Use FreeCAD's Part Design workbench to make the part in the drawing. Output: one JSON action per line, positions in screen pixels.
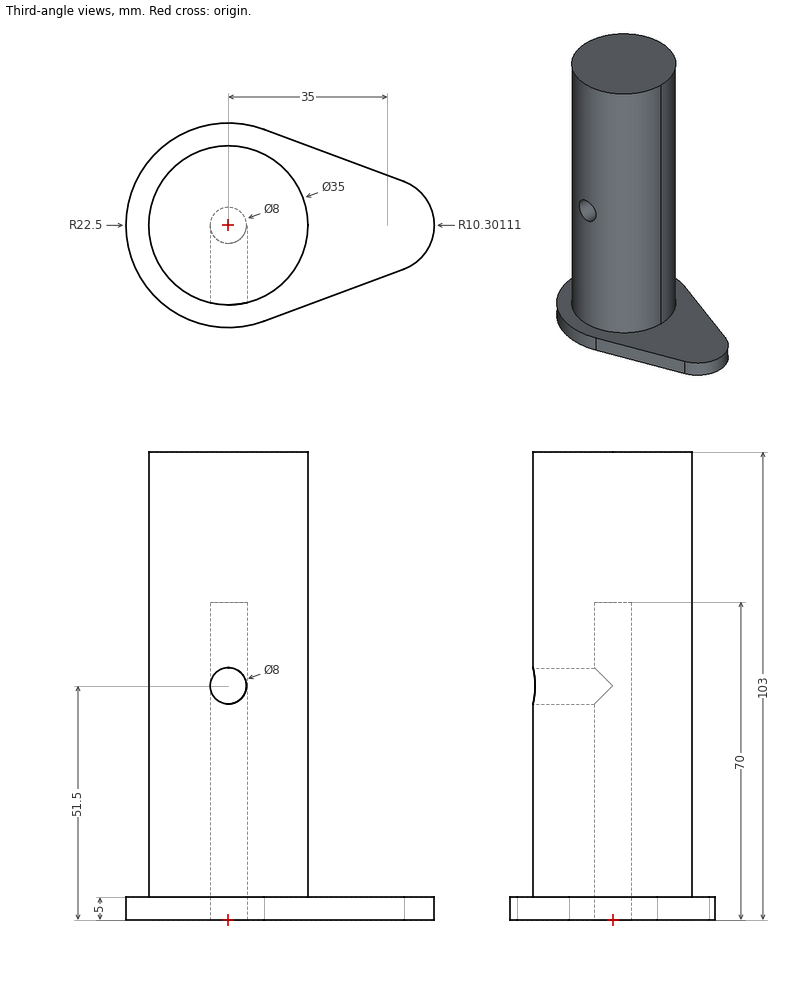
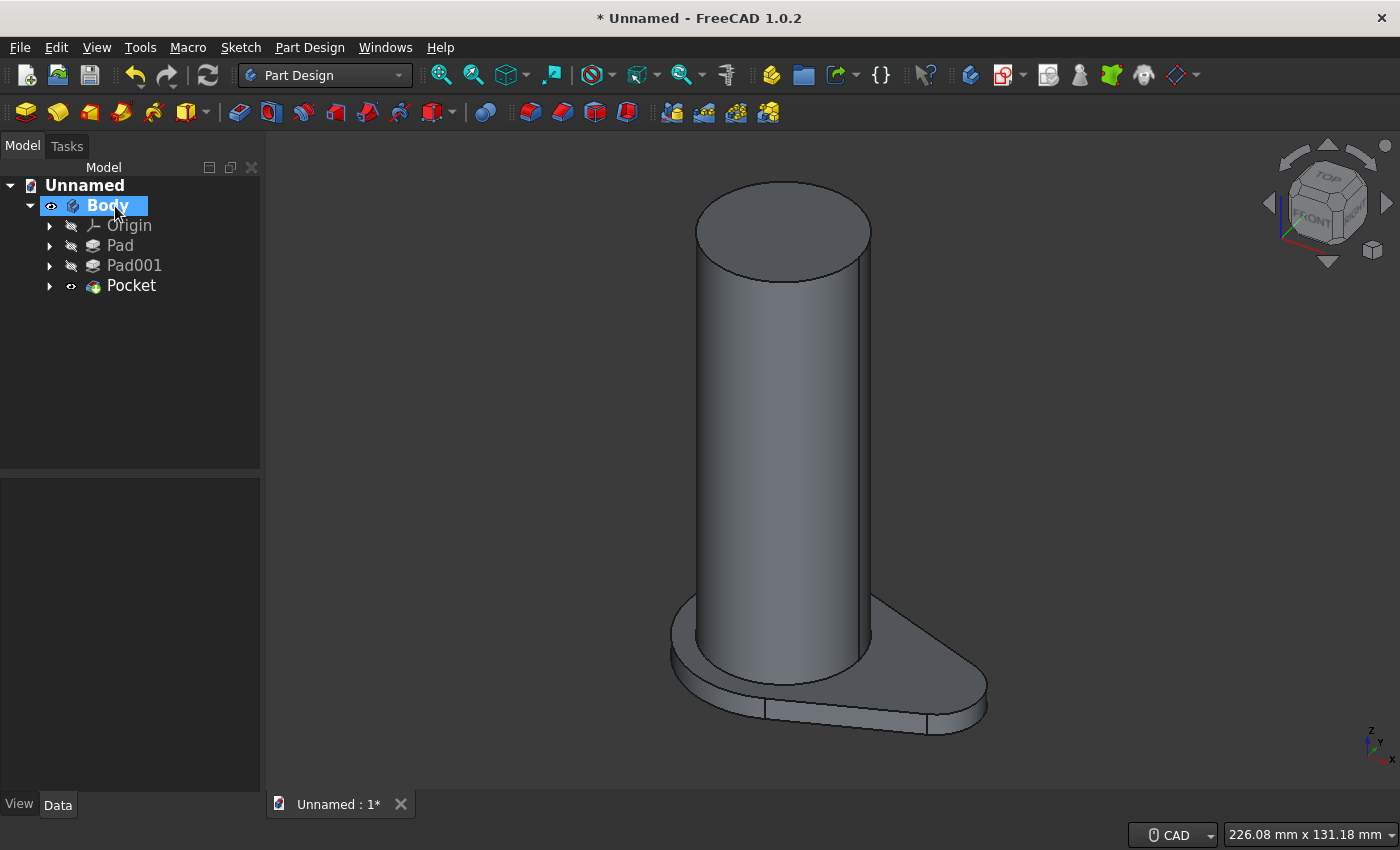
{"action": "left_click", "coordinate": [1004, 76]}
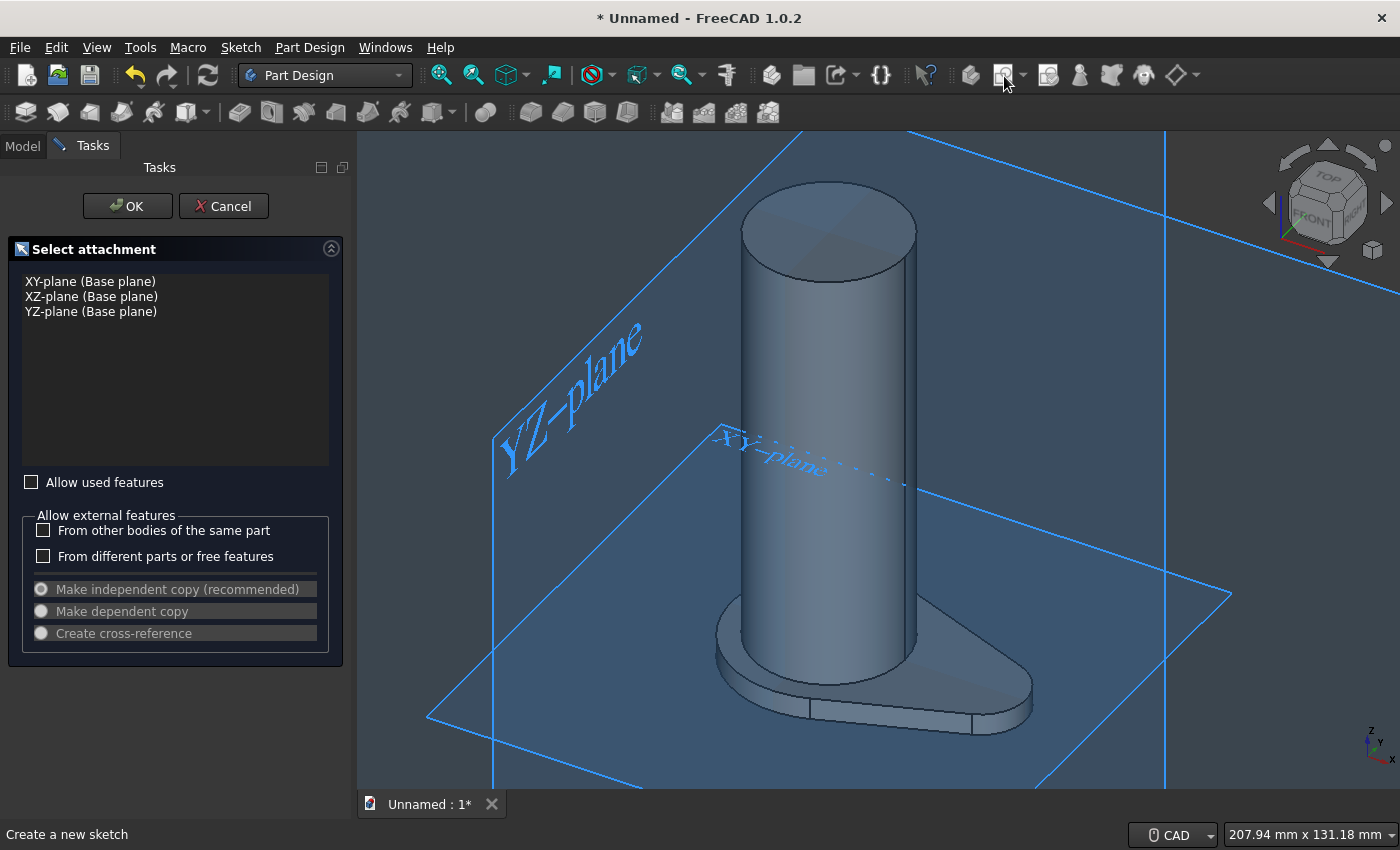
{"action": "left_click", "coordinate": [82, 296]}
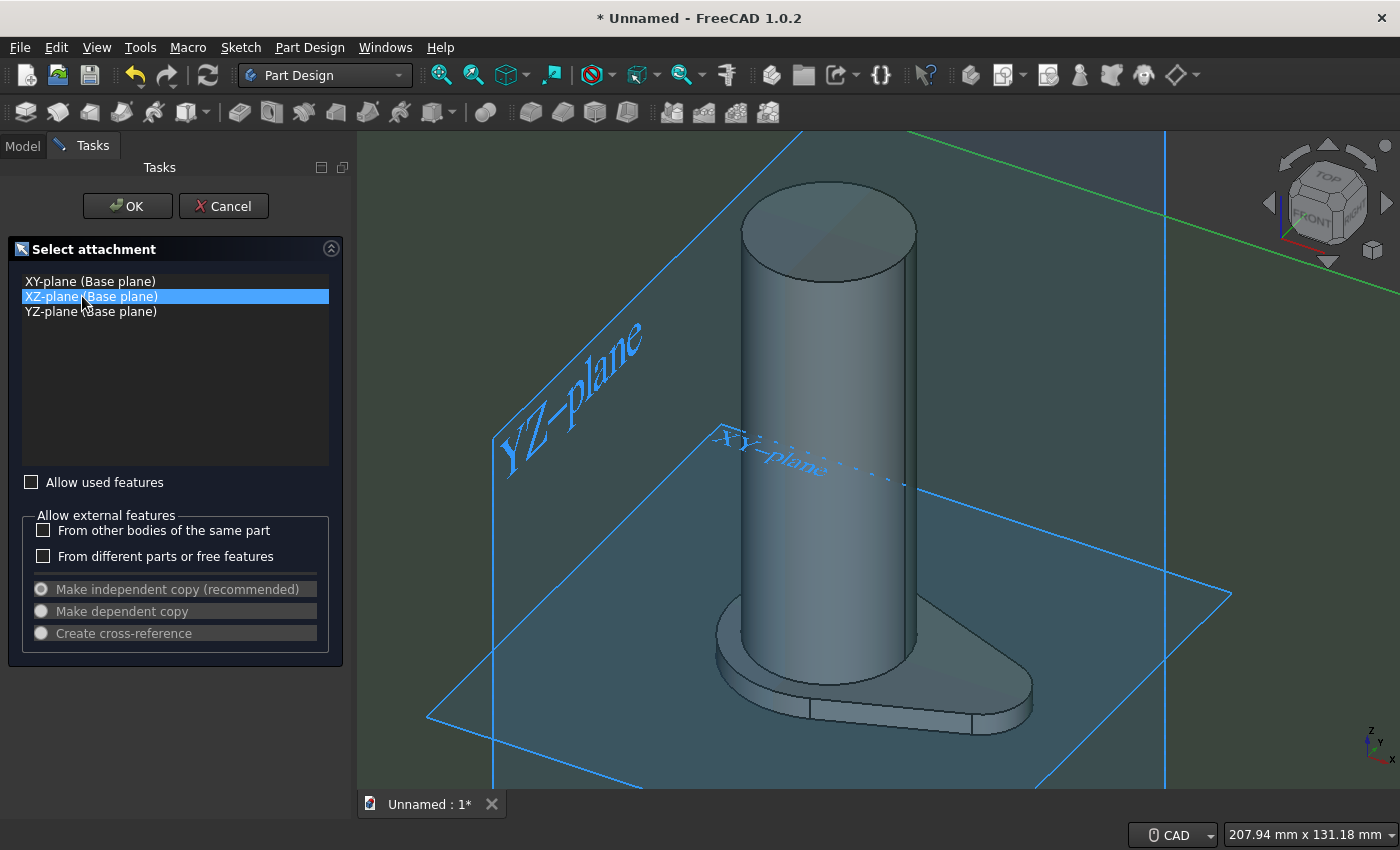
{"action": "left_click", "coordinate": [128, 206]}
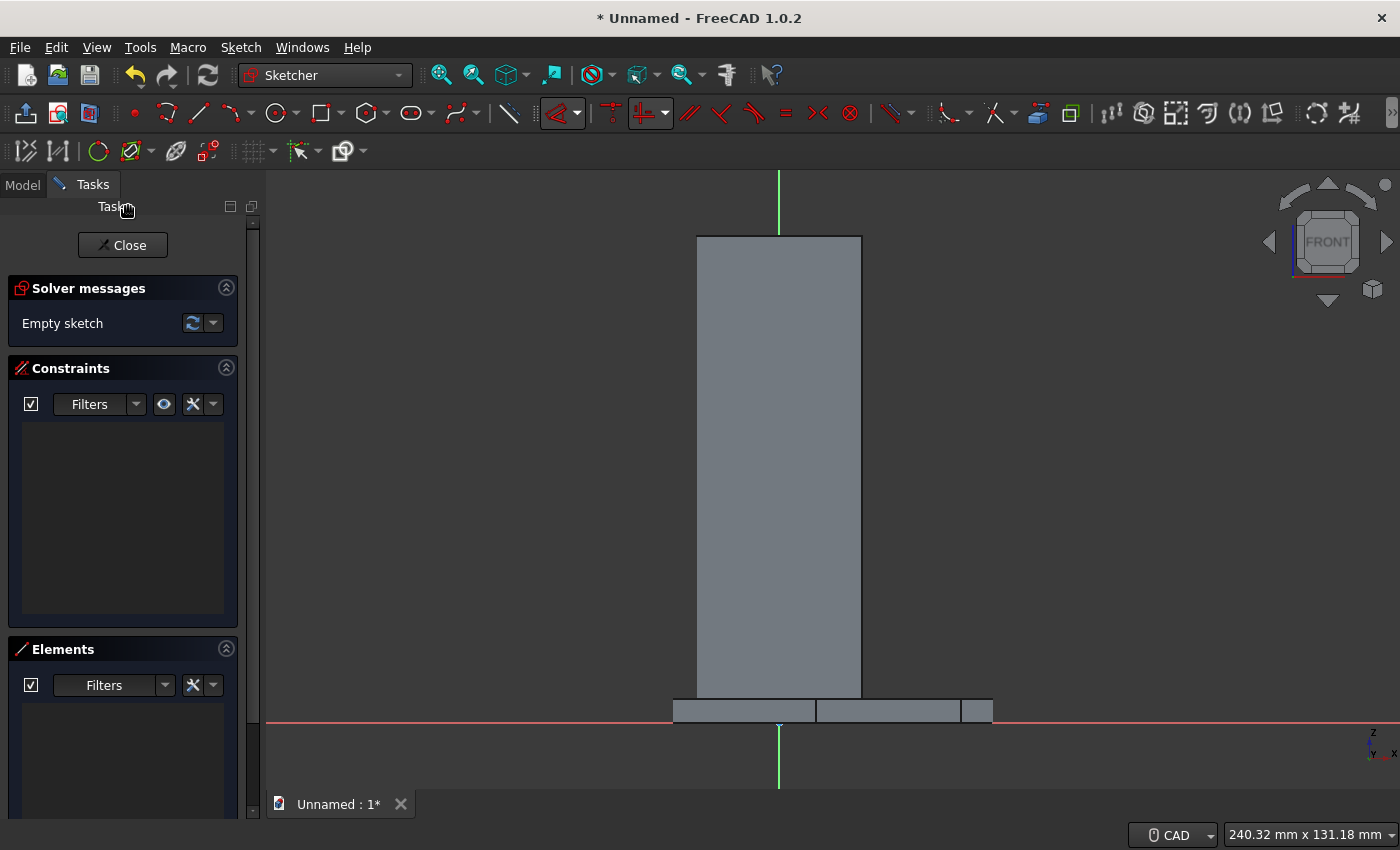
{"action": "left_click", "coordinate": [90, 114]}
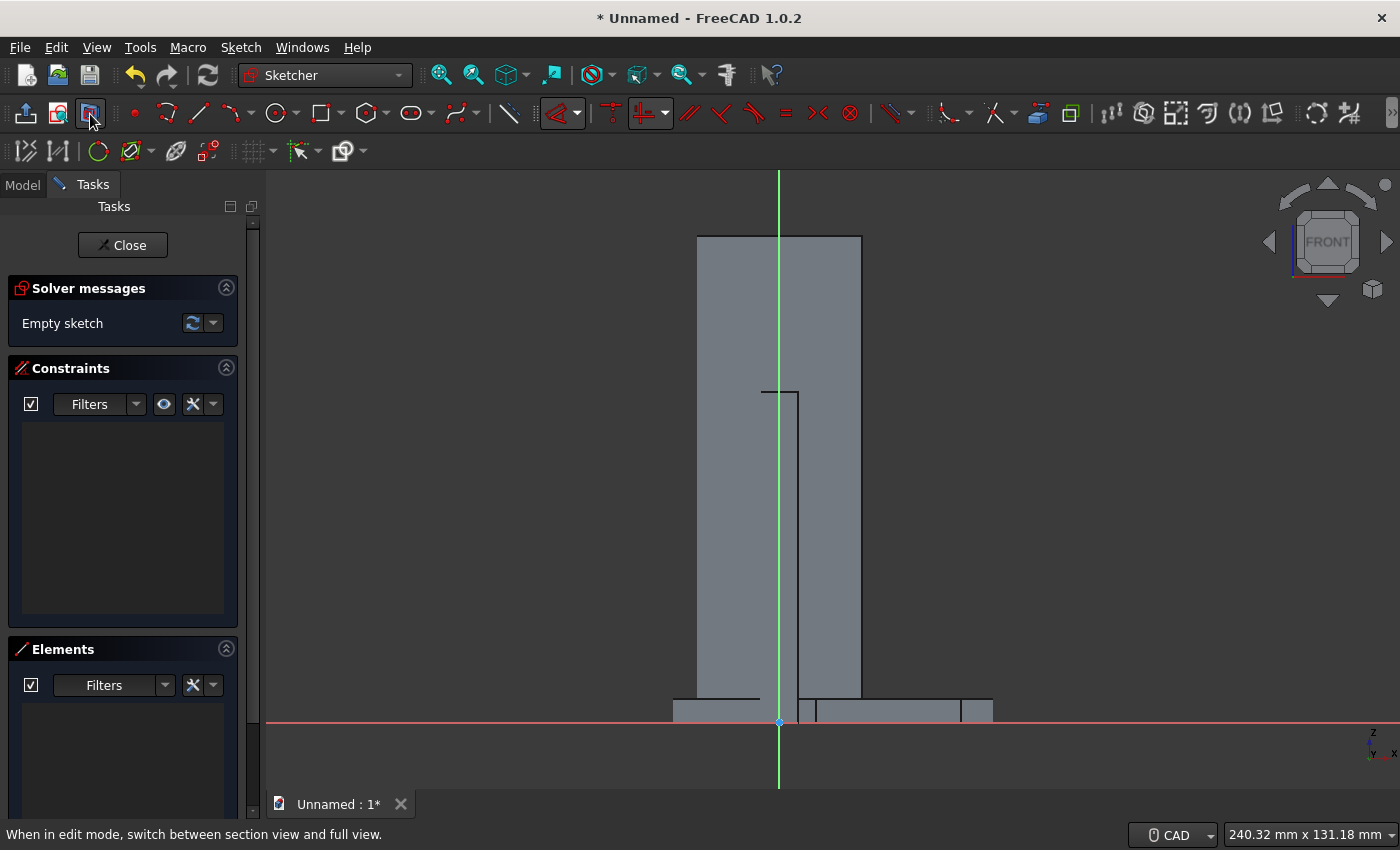
{"action": "scroll", "coordinate": [781, 480], "scroll_direction": "up", "scroll_amount": 12}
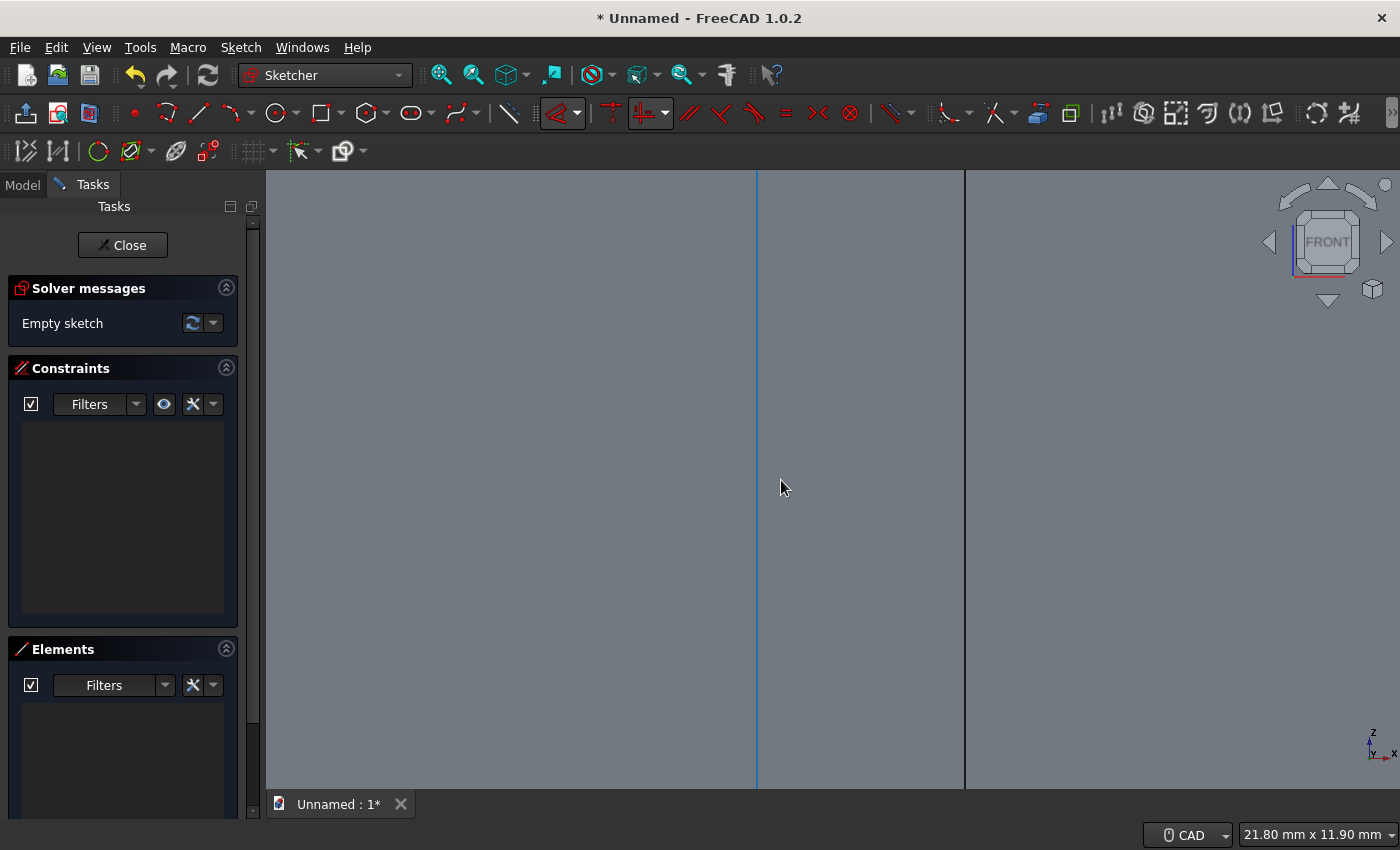
{"action": "left_click", "coordinate": [276, 114]}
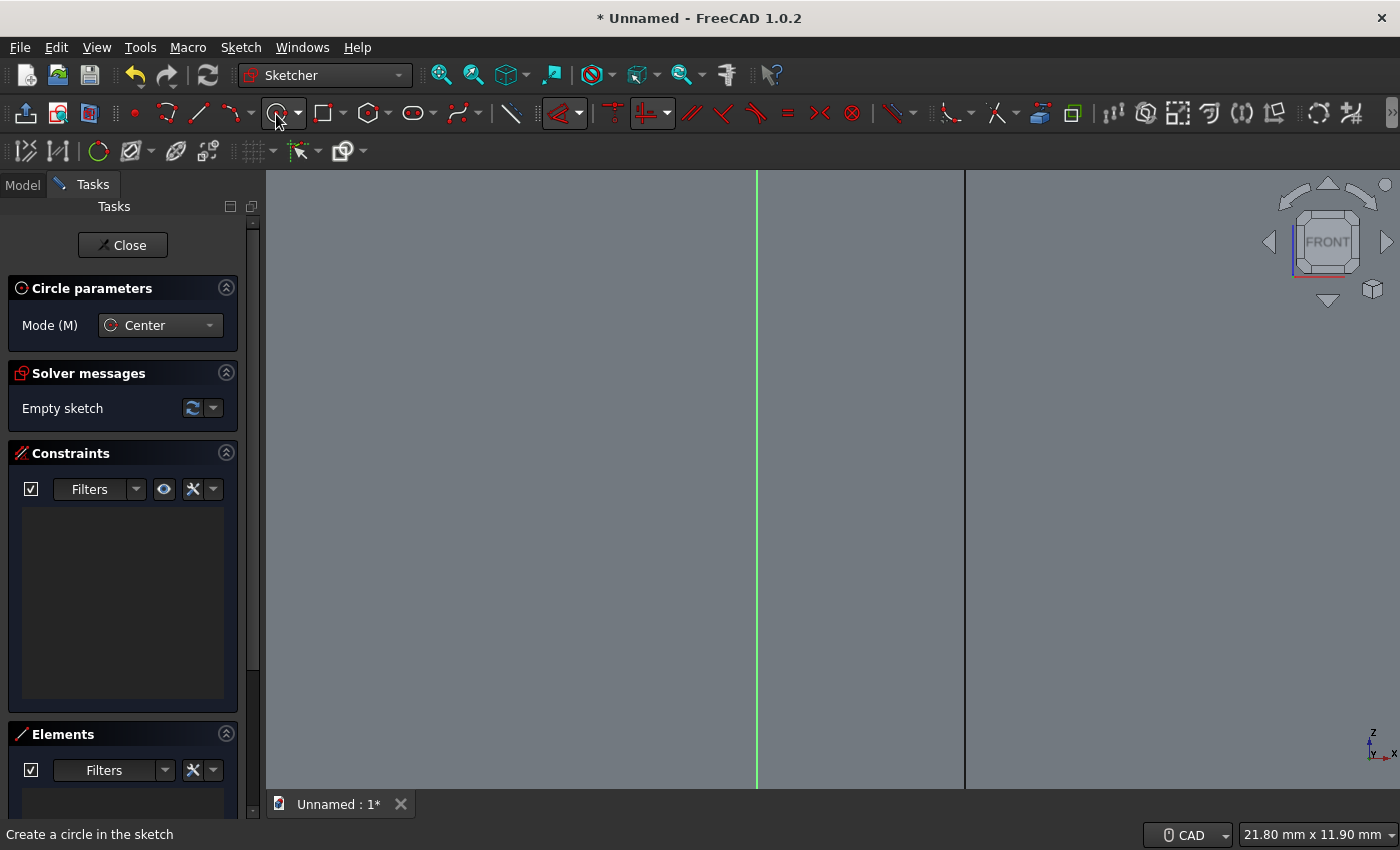
{"action": "left_click", "coordinate": [757, 469]}
{"action": "left_click", "coordinate": [904, 322]}
{"action": "key", "text": "Escape"}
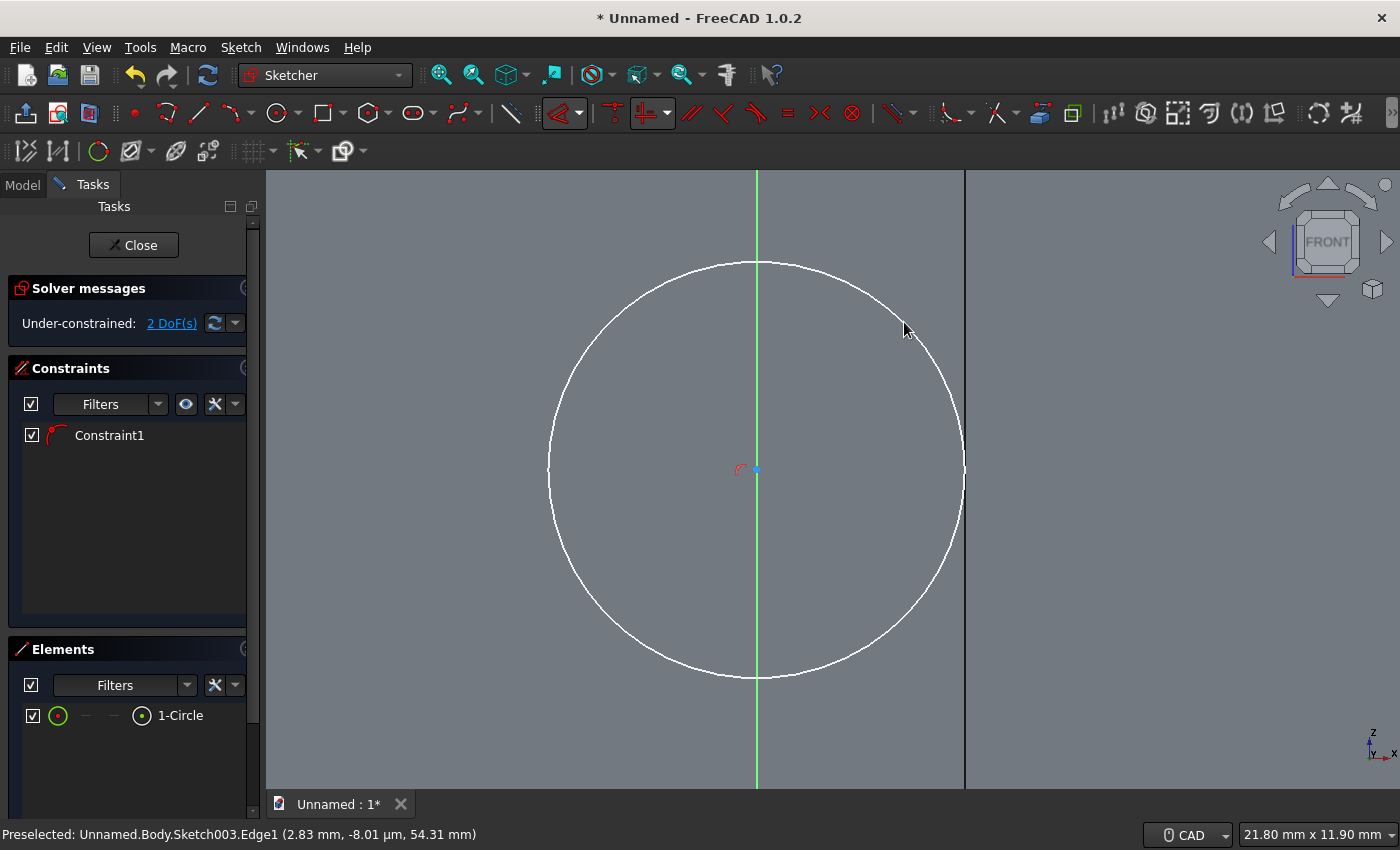
{"action": "left_click", "coordinate": [903, 322]}